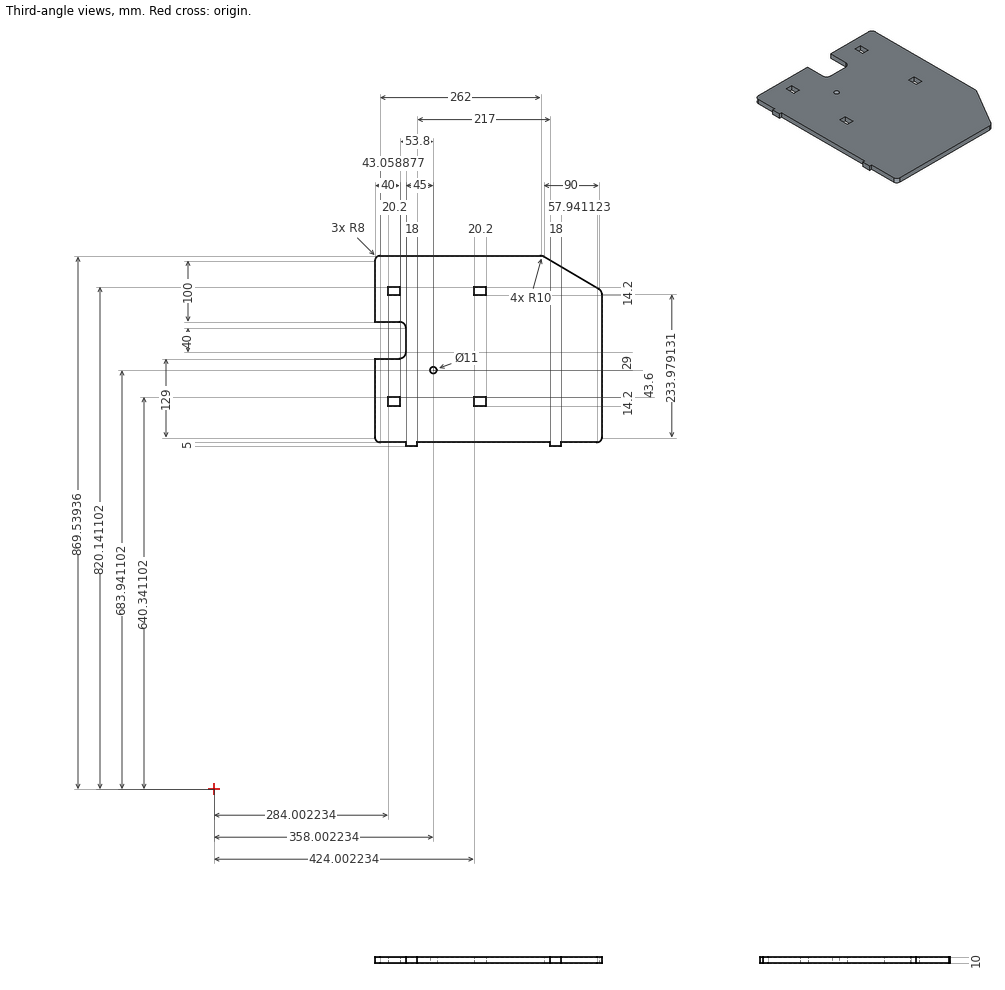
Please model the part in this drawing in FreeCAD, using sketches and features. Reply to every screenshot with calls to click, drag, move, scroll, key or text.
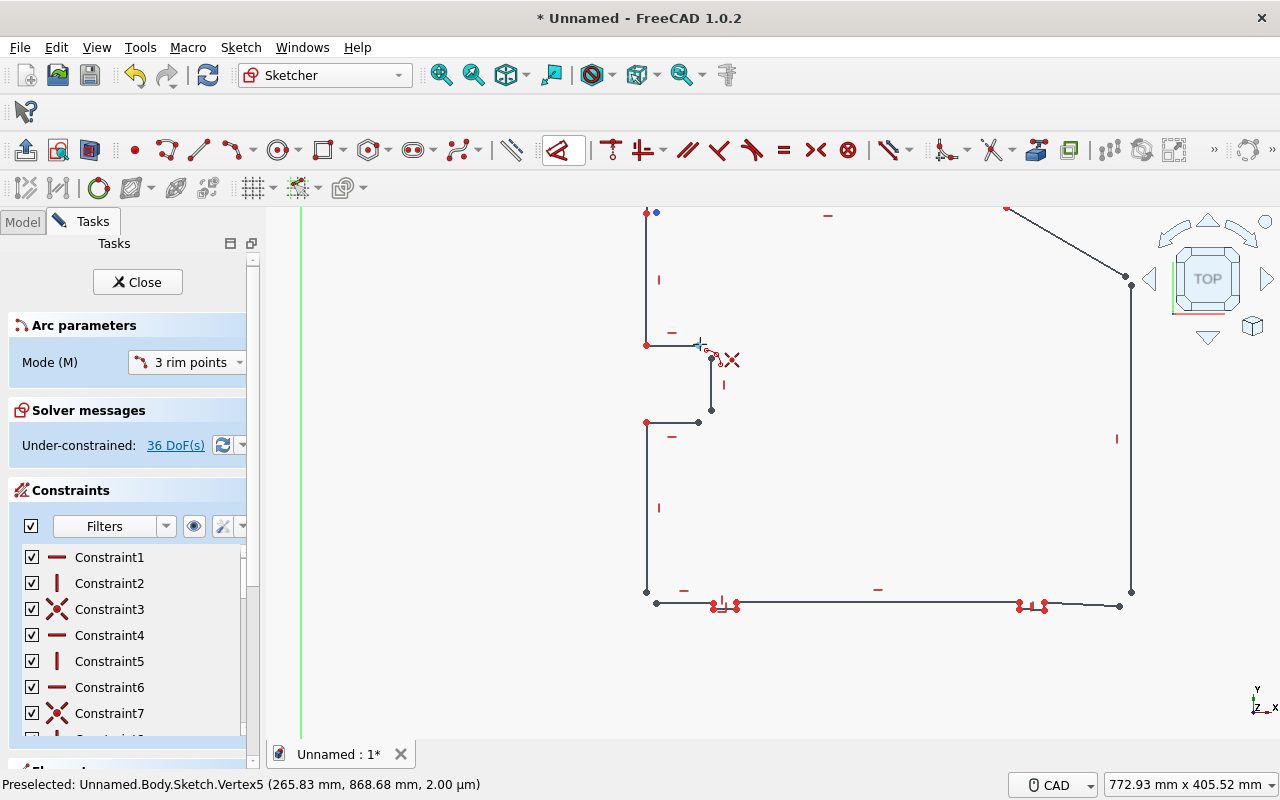
click(698, 346)
click(711, 358)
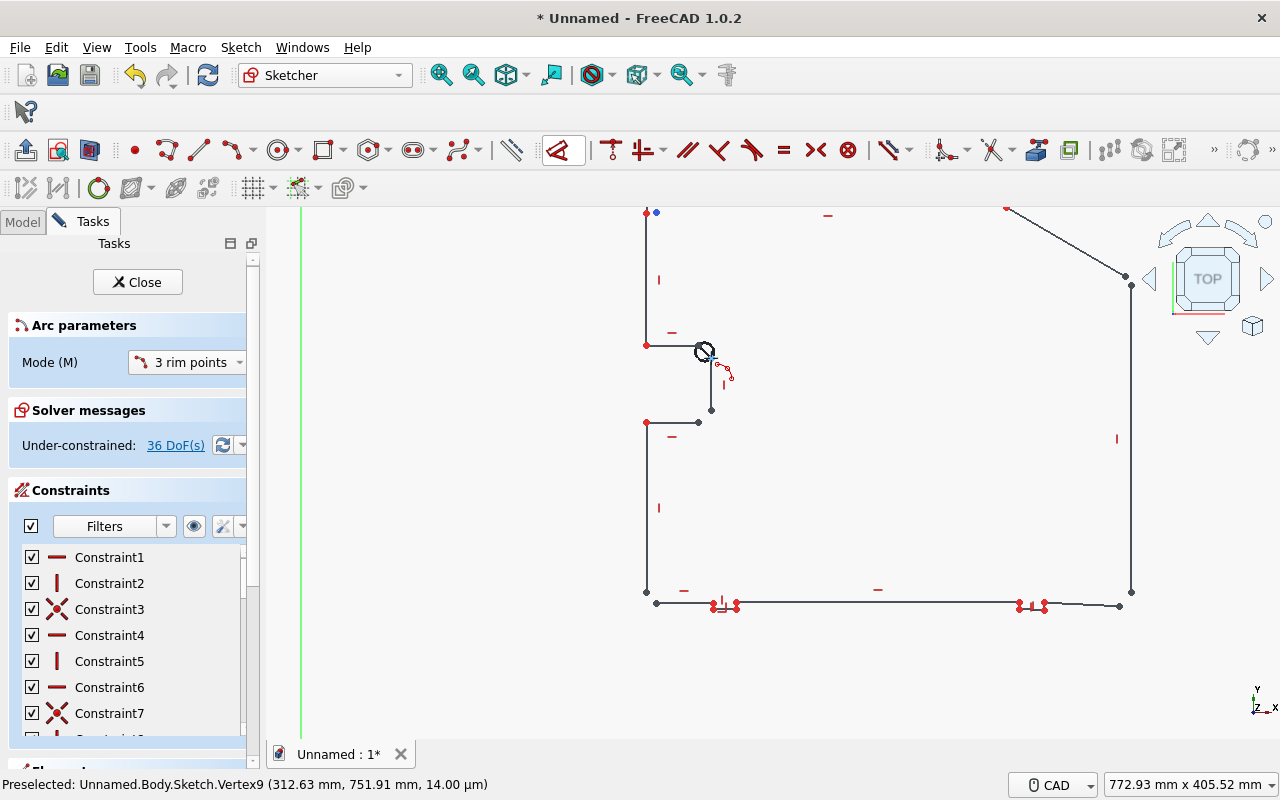
scroll(708, 348, up, 8)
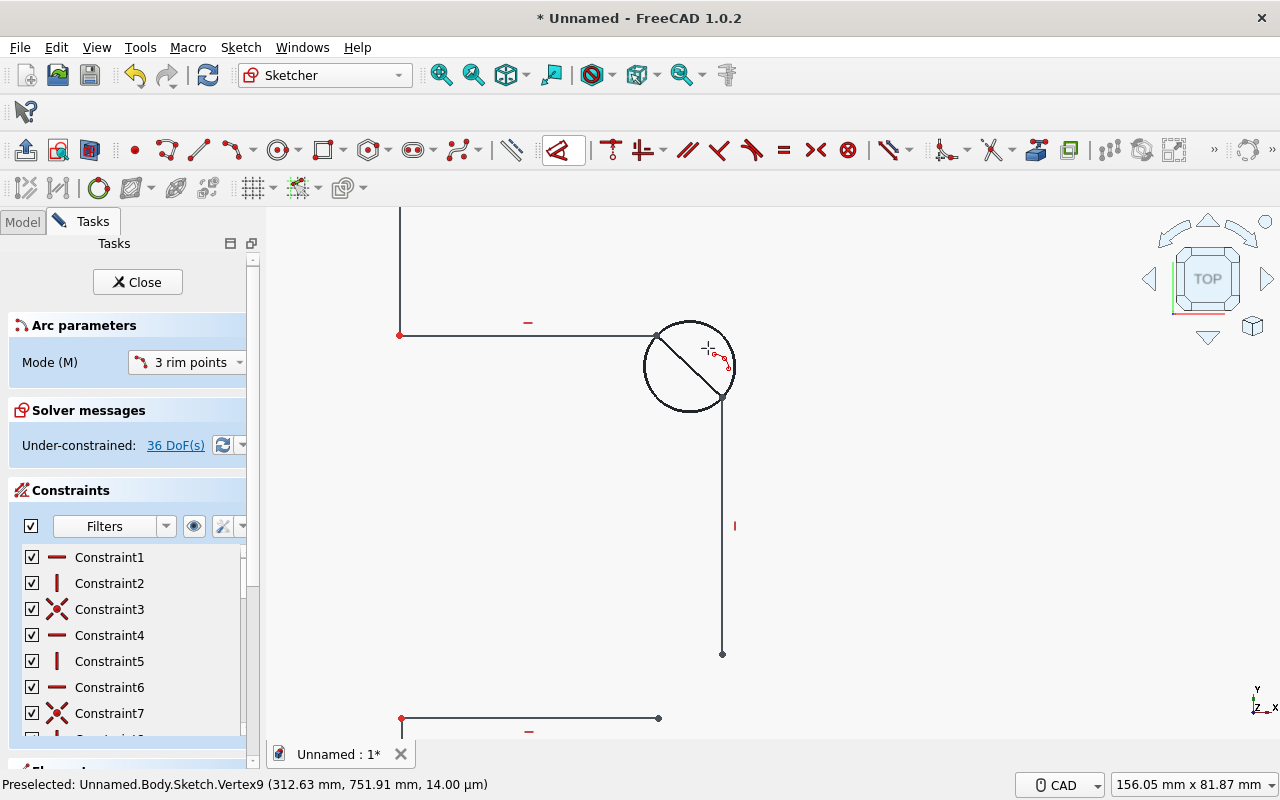
click(706, 345)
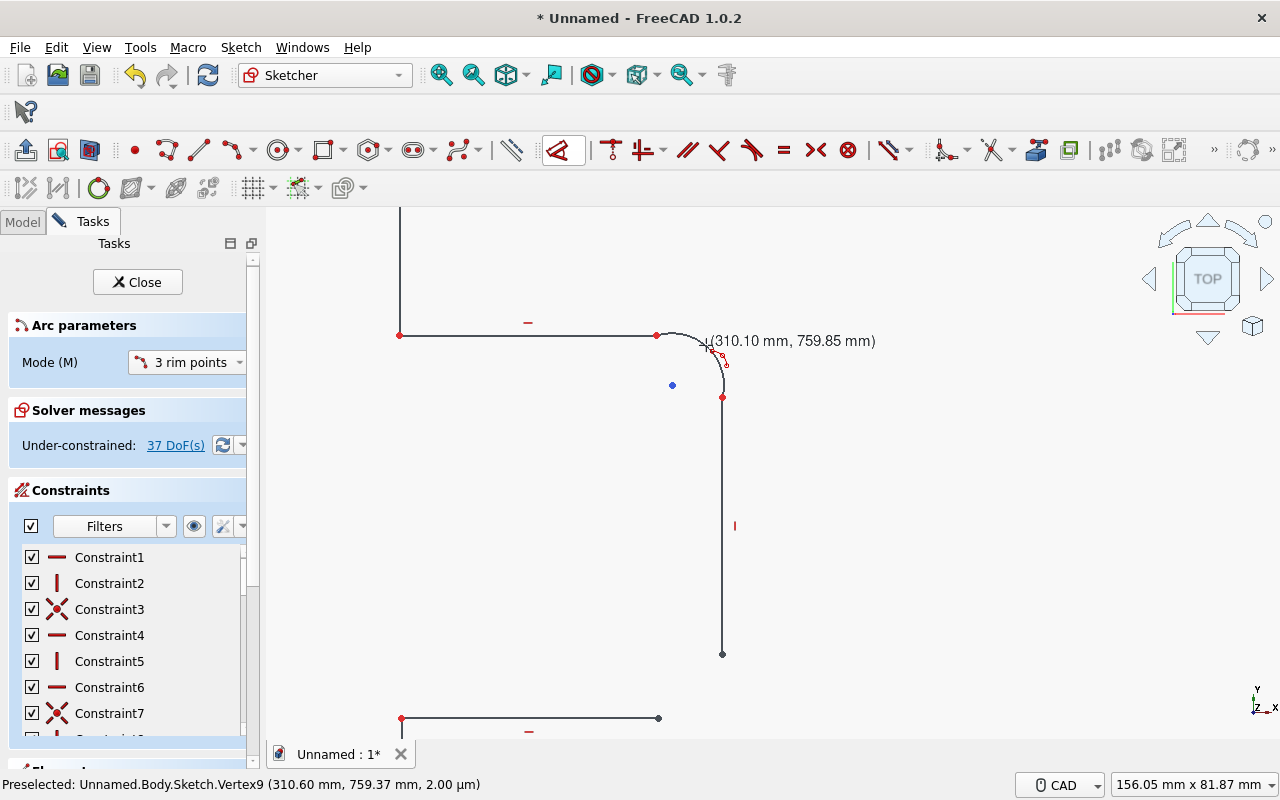
scroll(702, 345, down, 14)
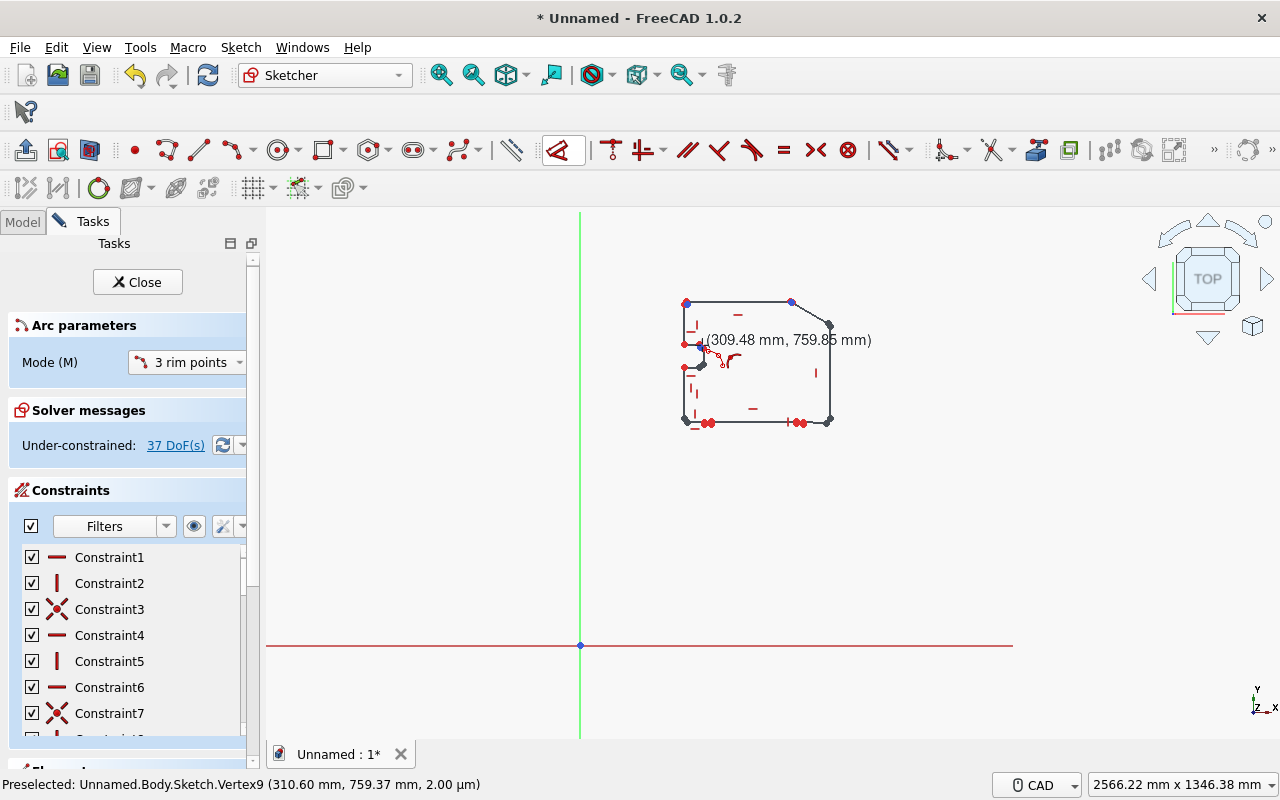
scroll(704, 364, up, 6)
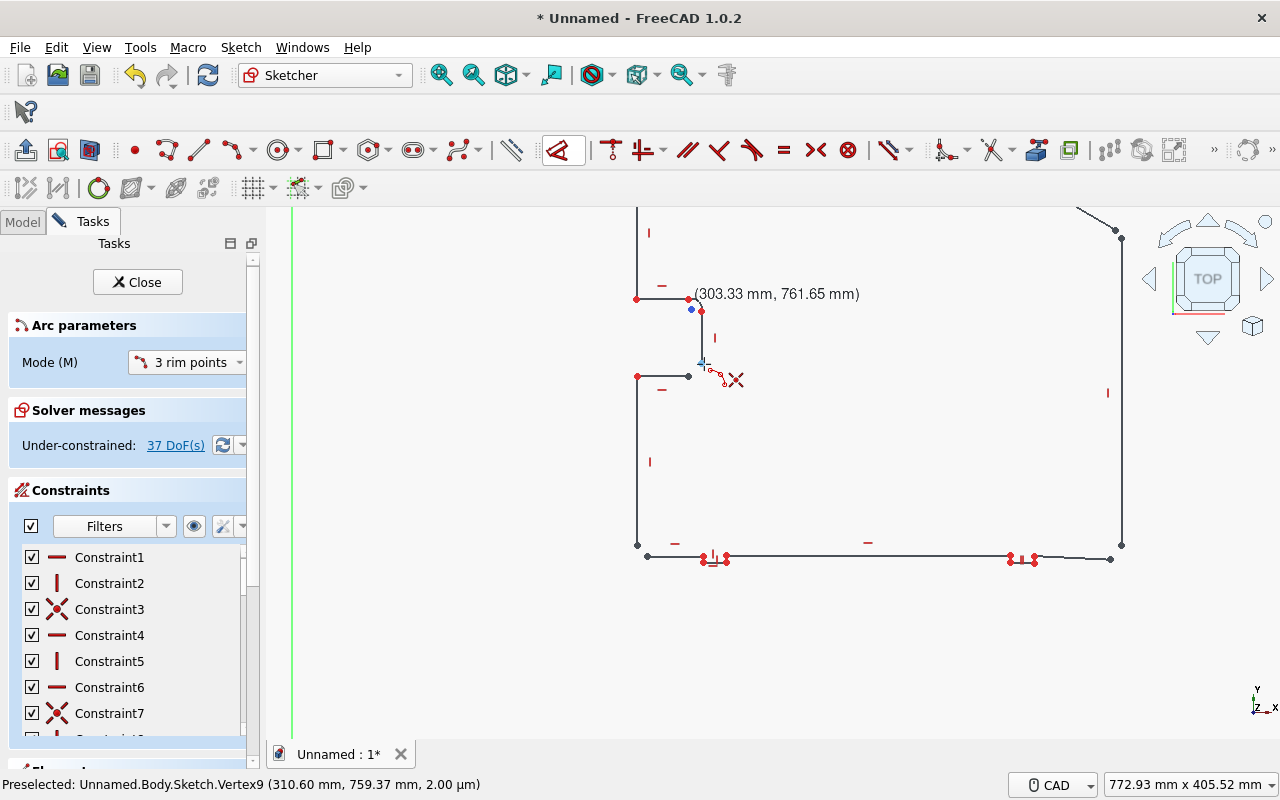
click(702, 363)
click(689, 376)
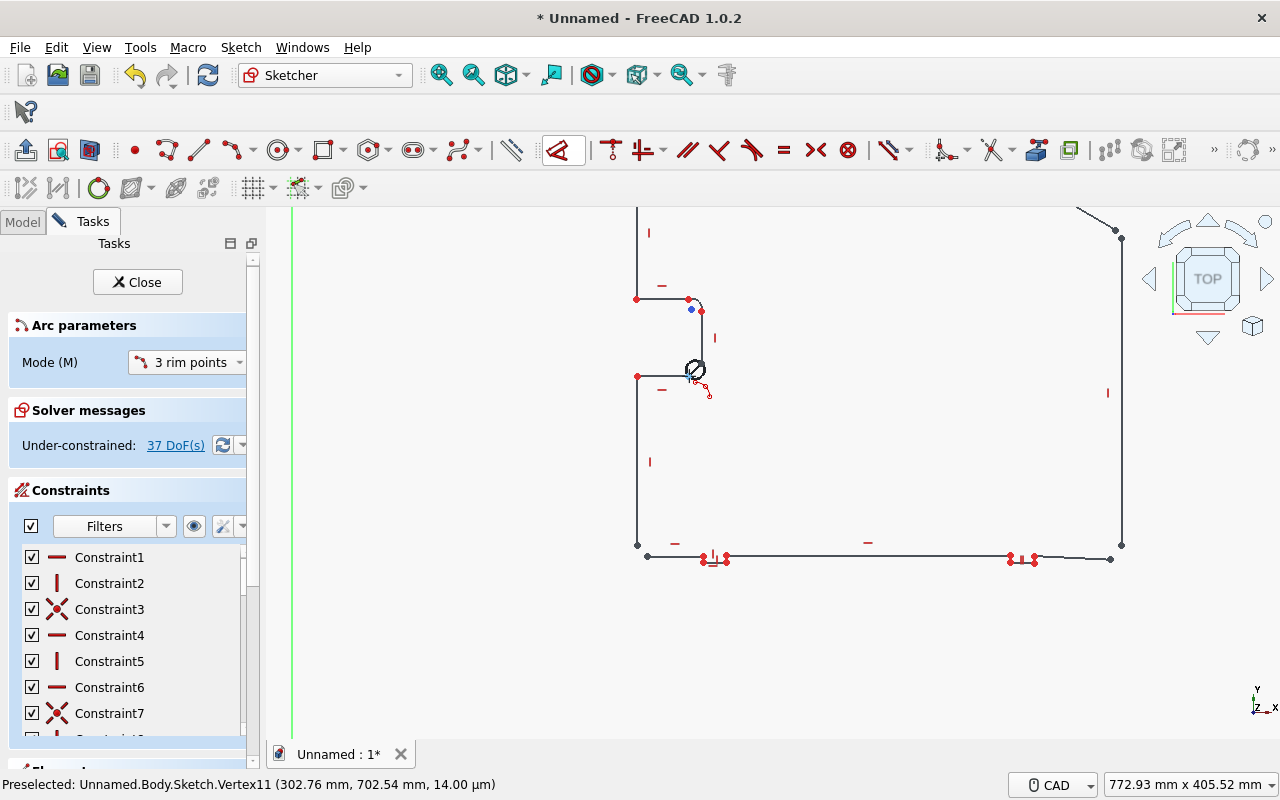
scroll(698, 372, up, 8)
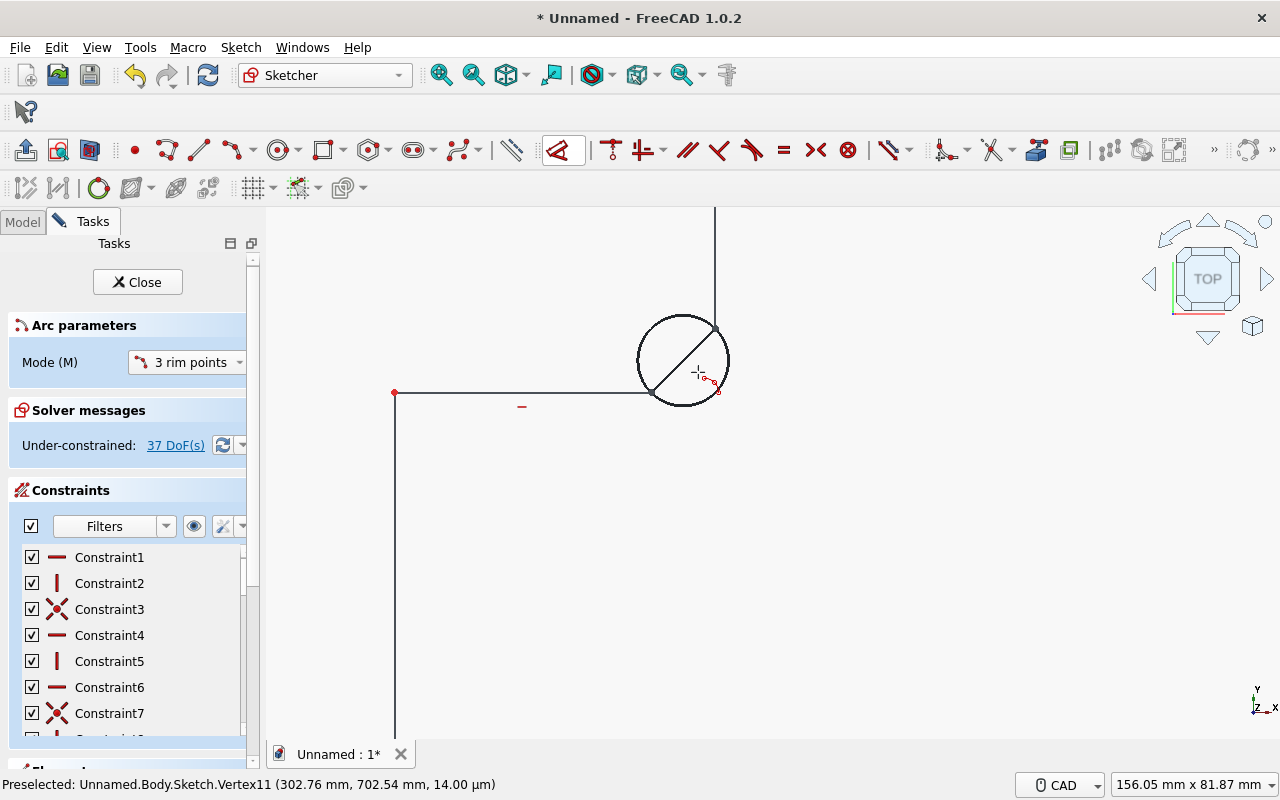
click(699, 371)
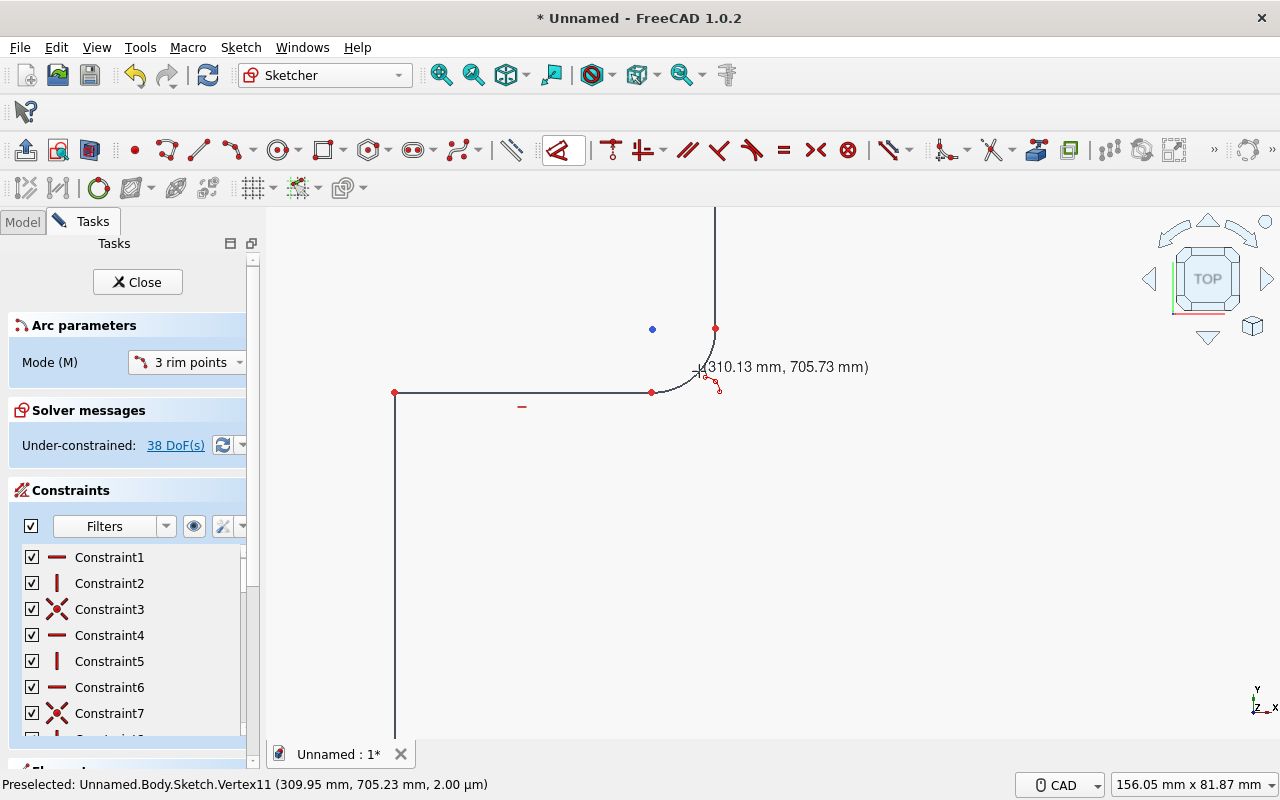
scroll(702, 366, down, 14)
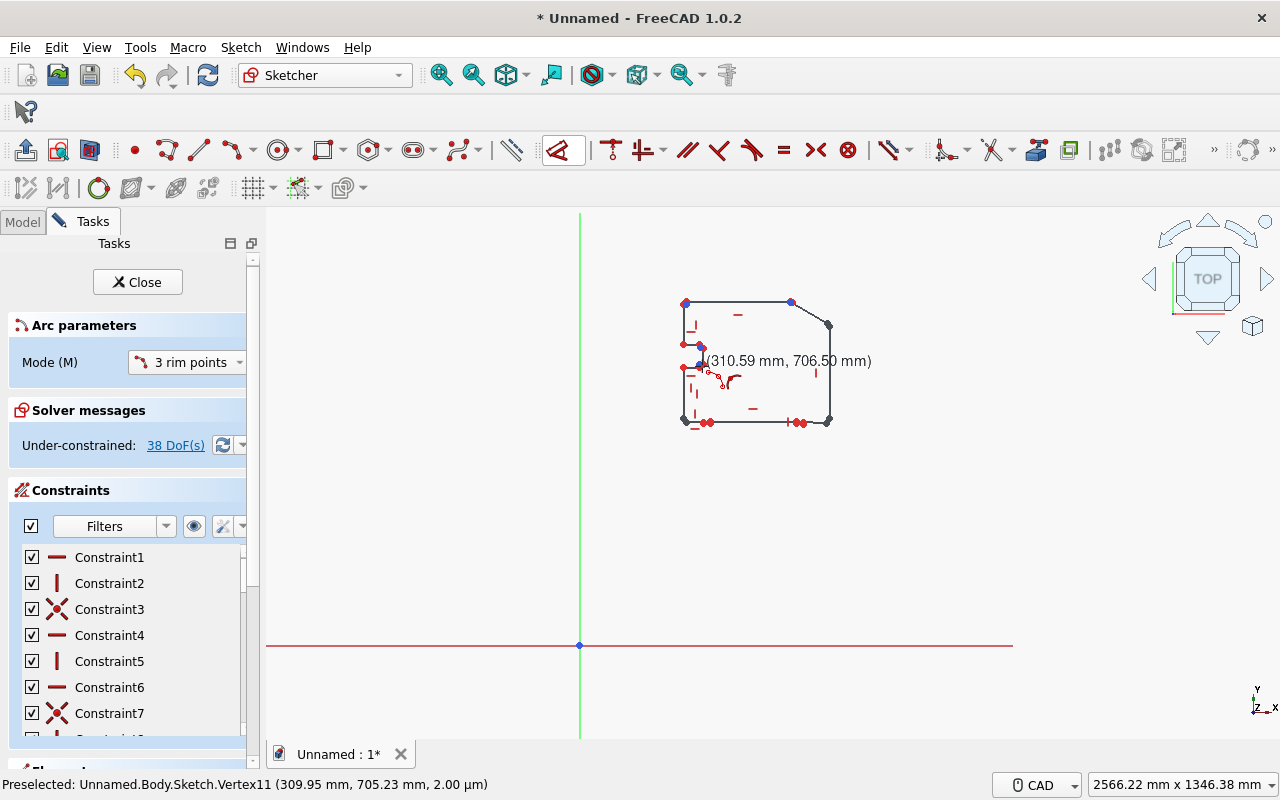
scroll(684, 419, up, 7)